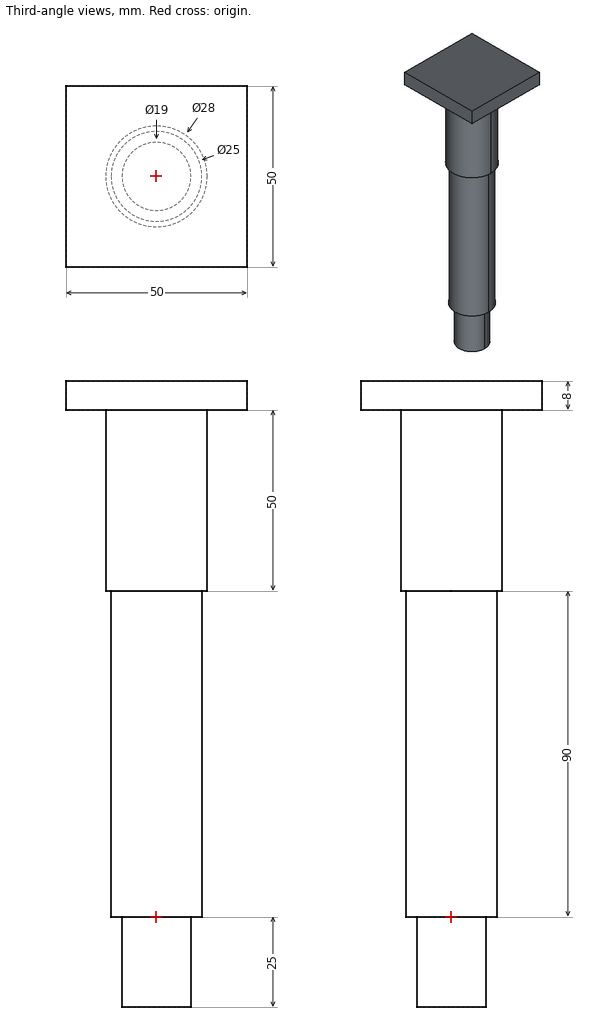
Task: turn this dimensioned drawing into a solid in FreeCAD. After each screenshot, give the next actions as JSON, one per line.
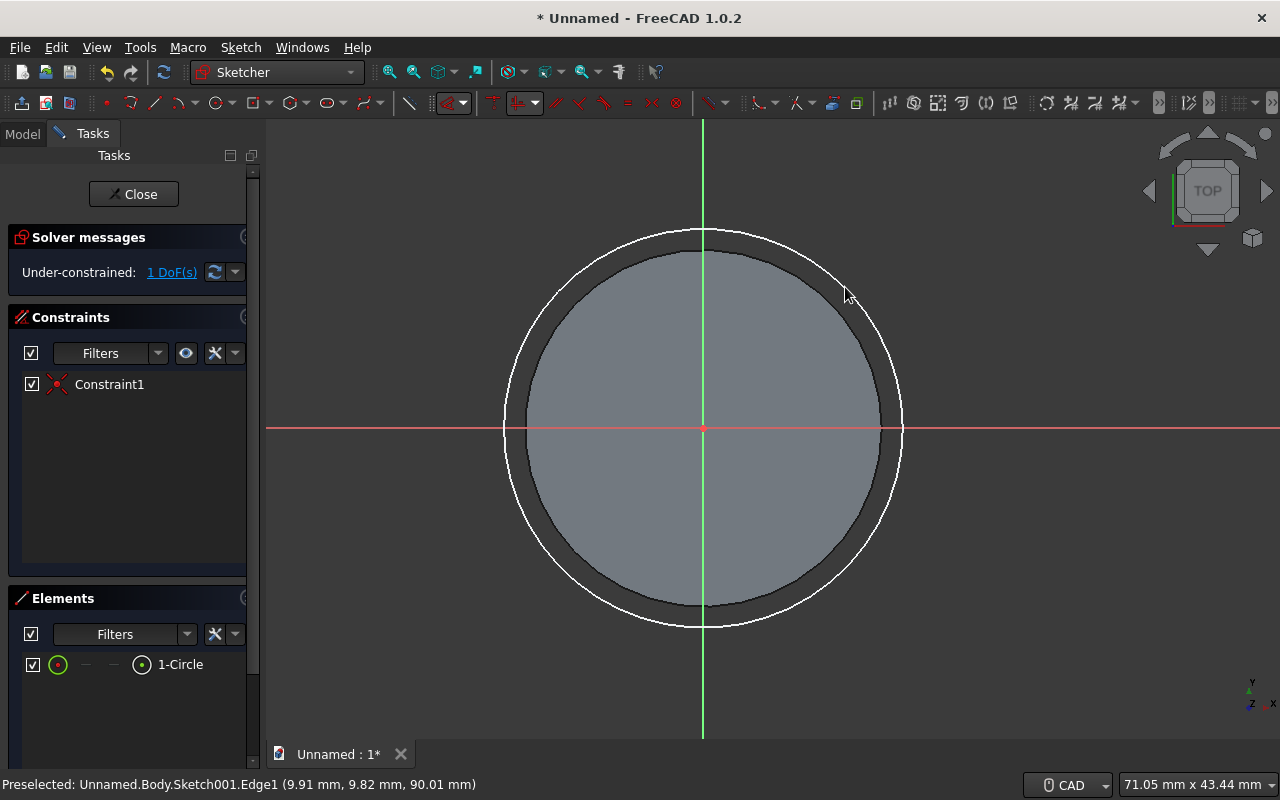
{"action": "key", "text": "d"}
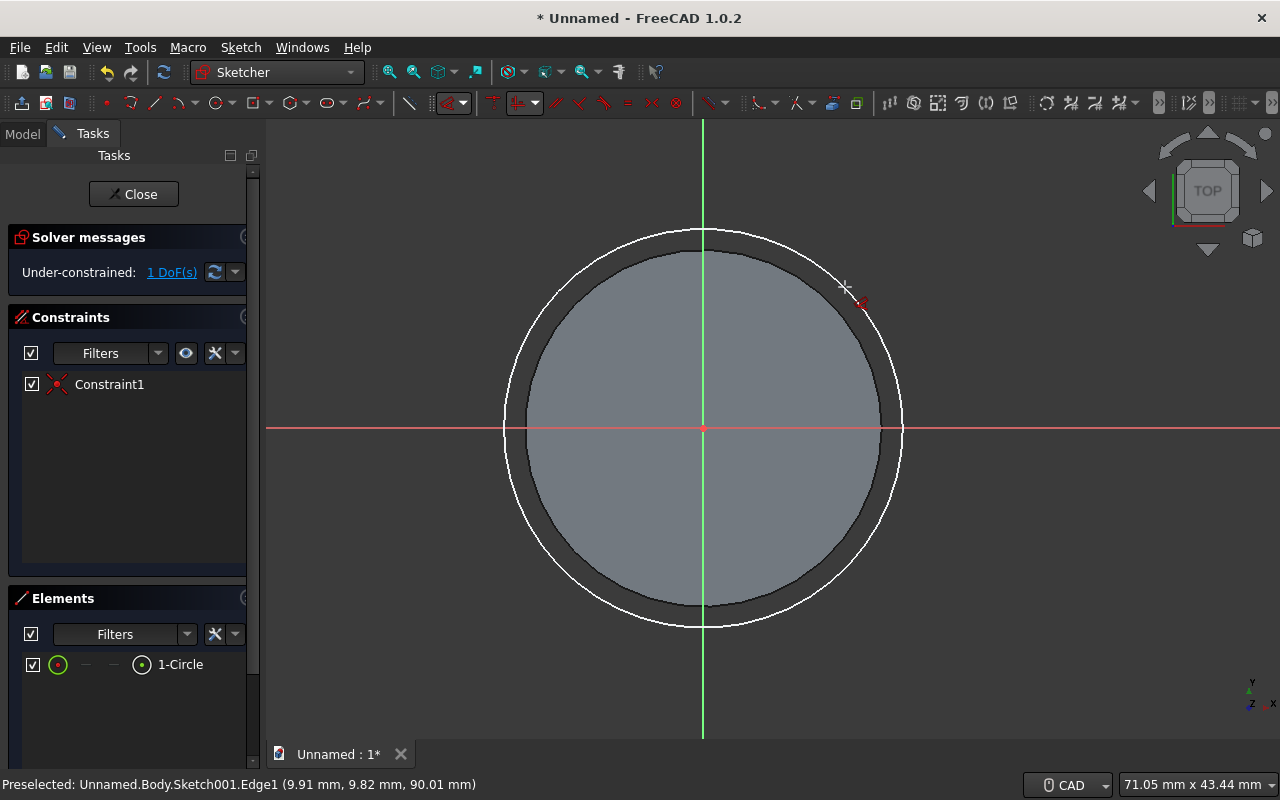
{"action": "left_click", "coordinate": [844, 287]}
{"action": "left_click", "coordinate": [867, 264]}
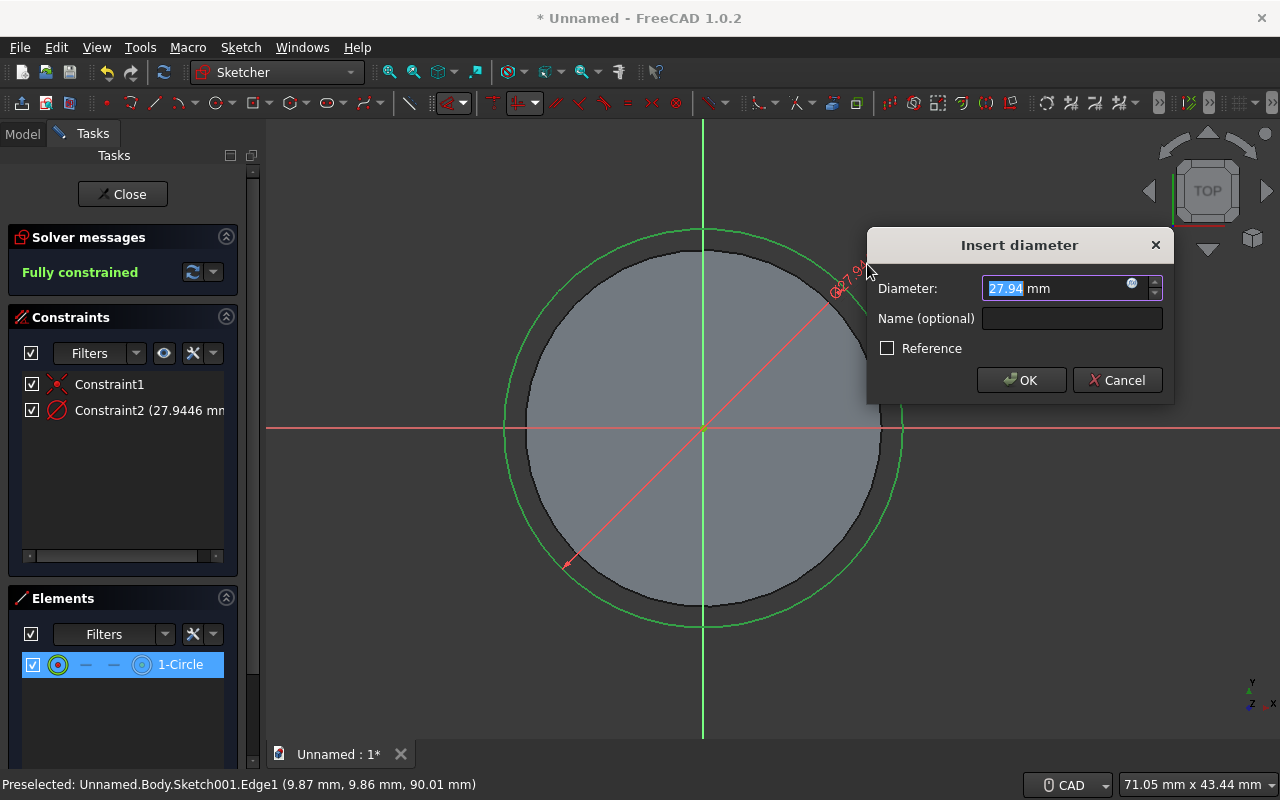
{"action": "type", "text": "28"}
{"action": "key", "text": "Return"}
{"action": "key", "text": "Escape"}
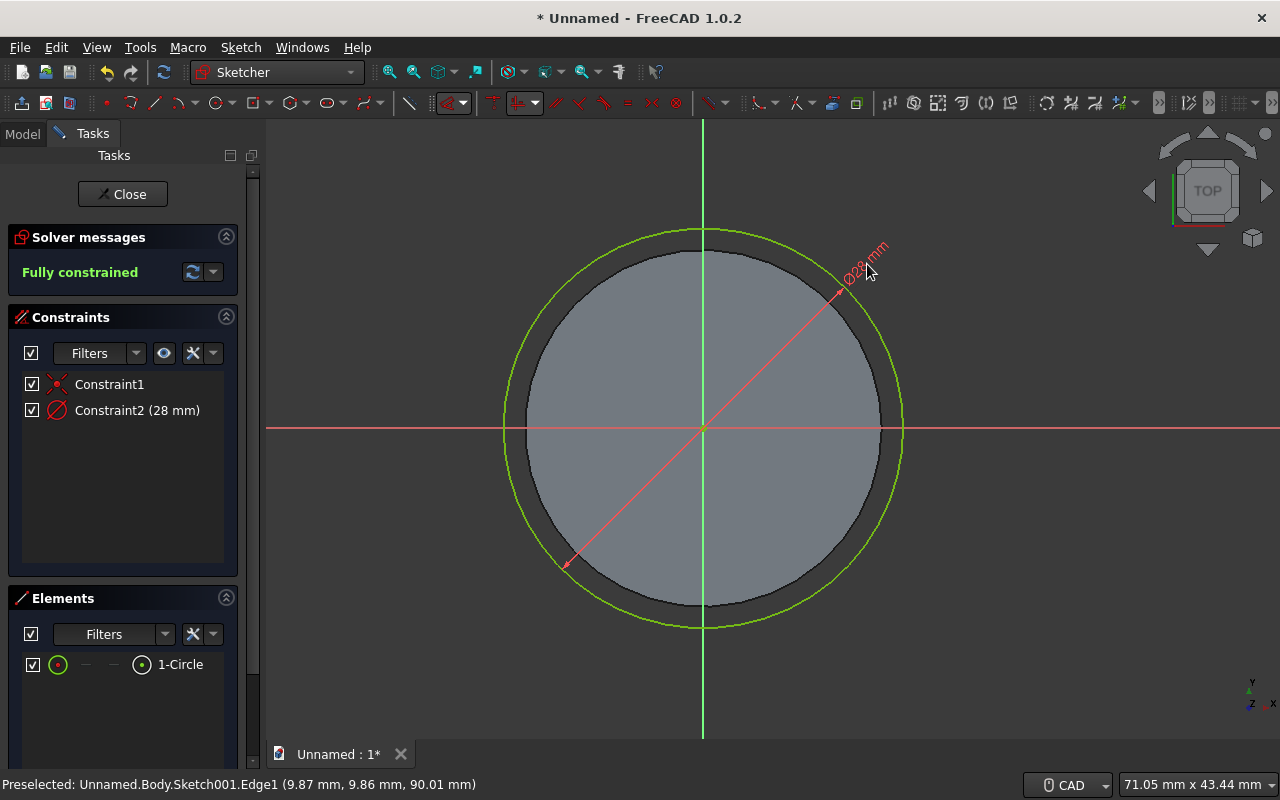
{"action": "left_click", "coordinate": [123, 194]}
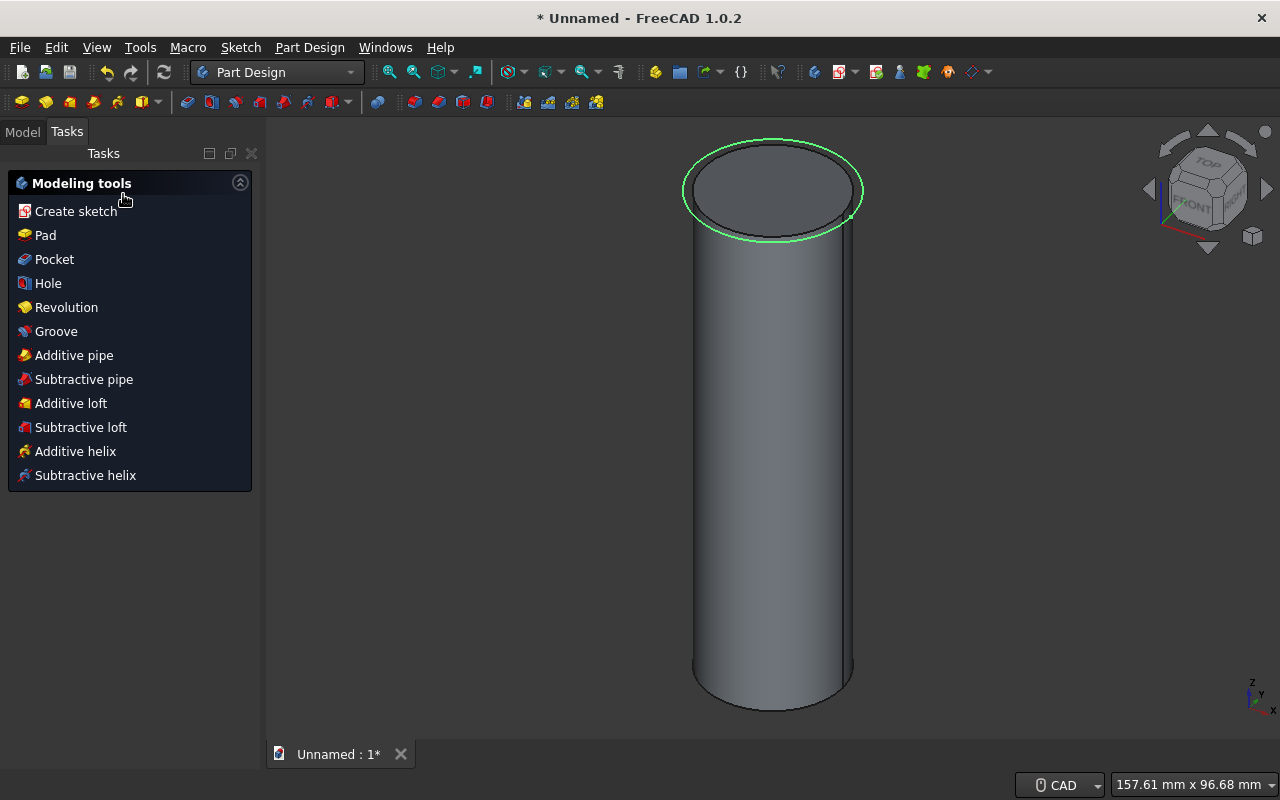
{"action": "left_click", "coordinate": [22, 102]}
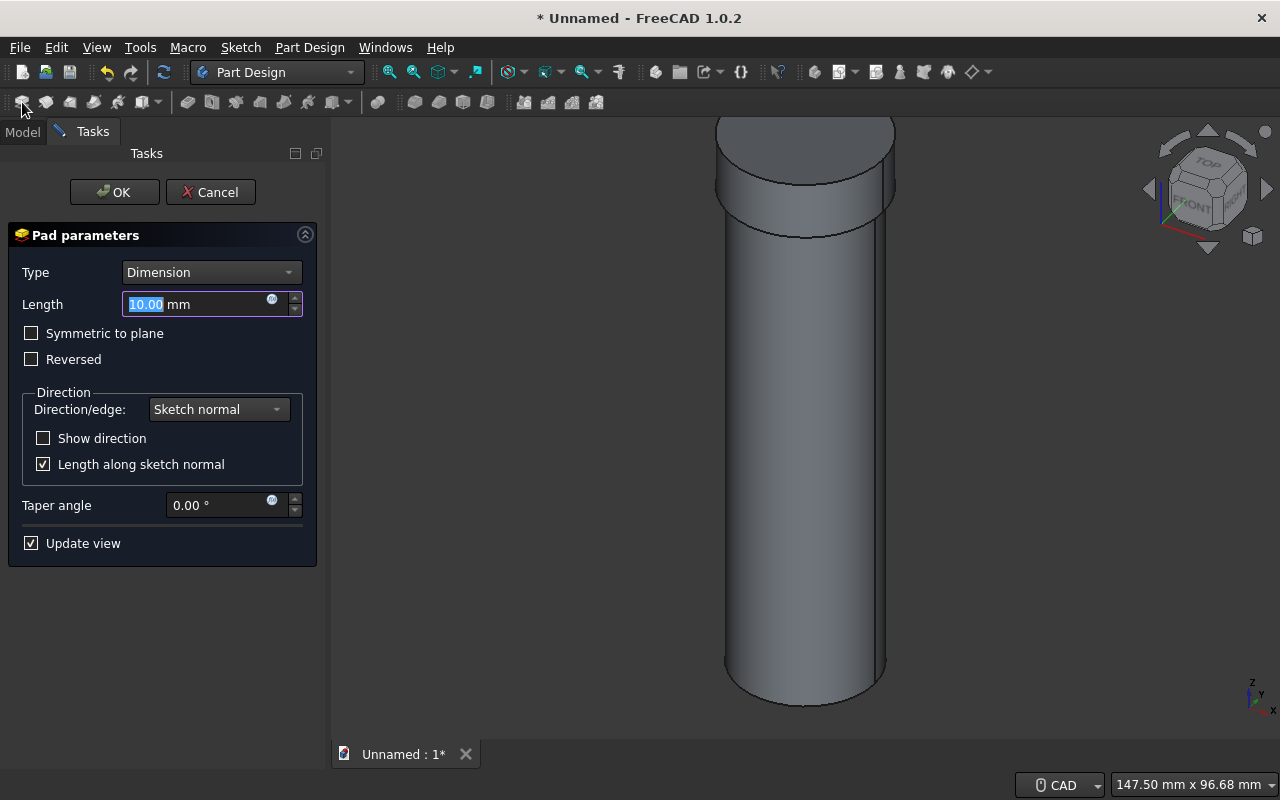
{"action": "type", "text": "50"}
{"action": "key", "text": "Tab"}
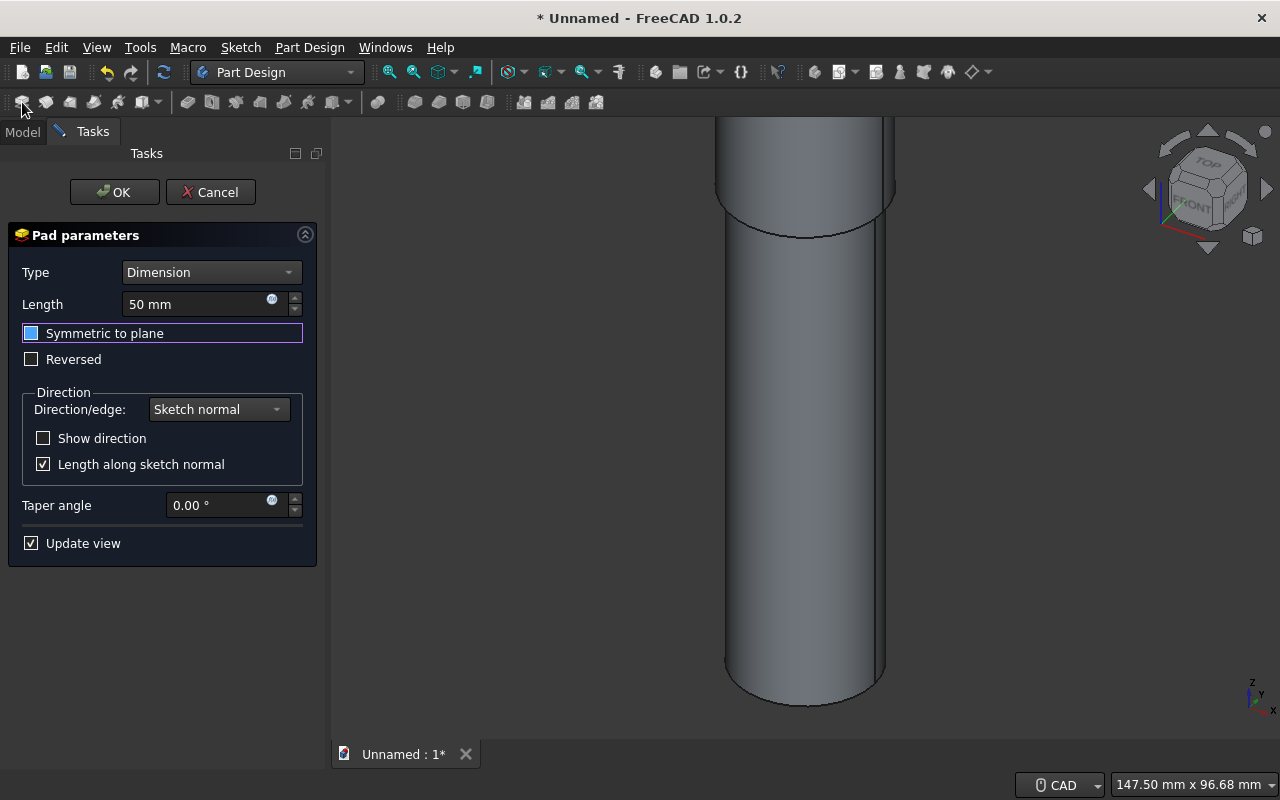
{"action": "left_click", "coordinate": [115, 192]}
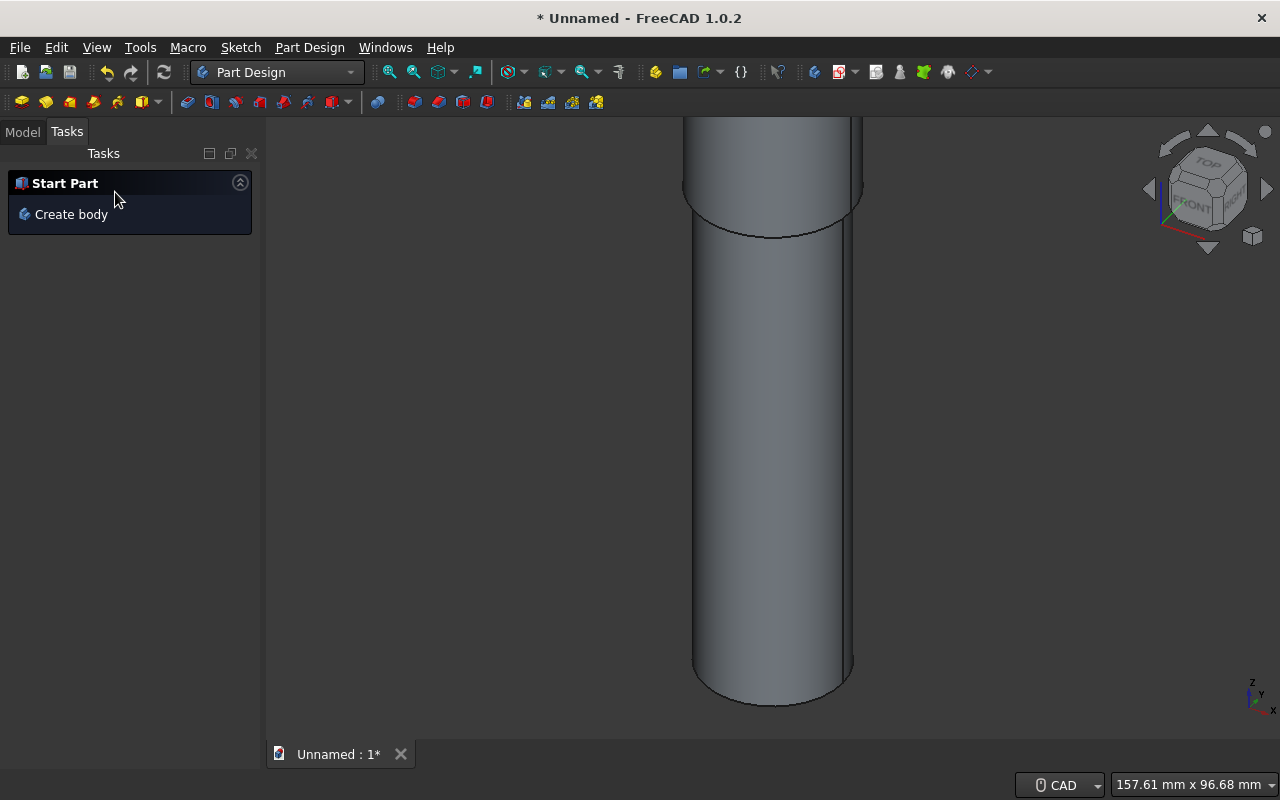
{"action": "key", "text": "v f"}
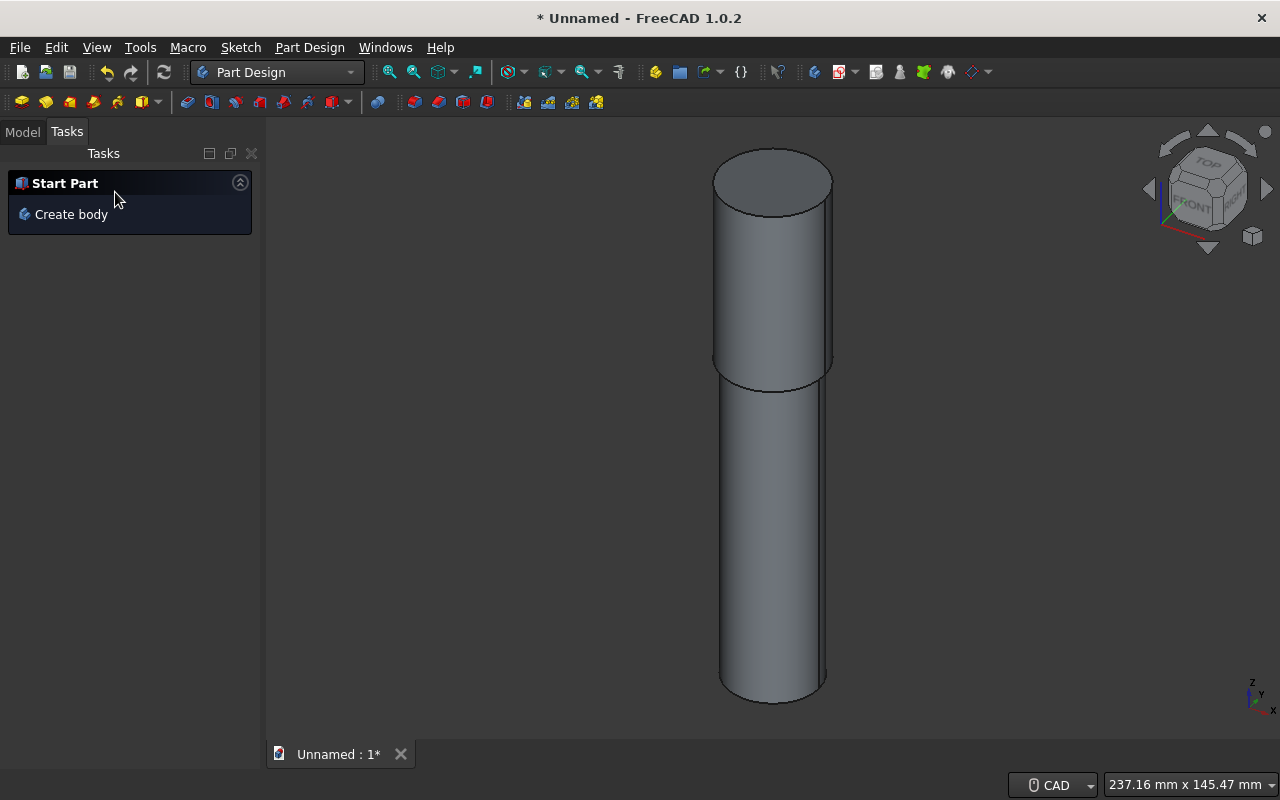
{"action": "left_click", "coordinate": [773, 182]}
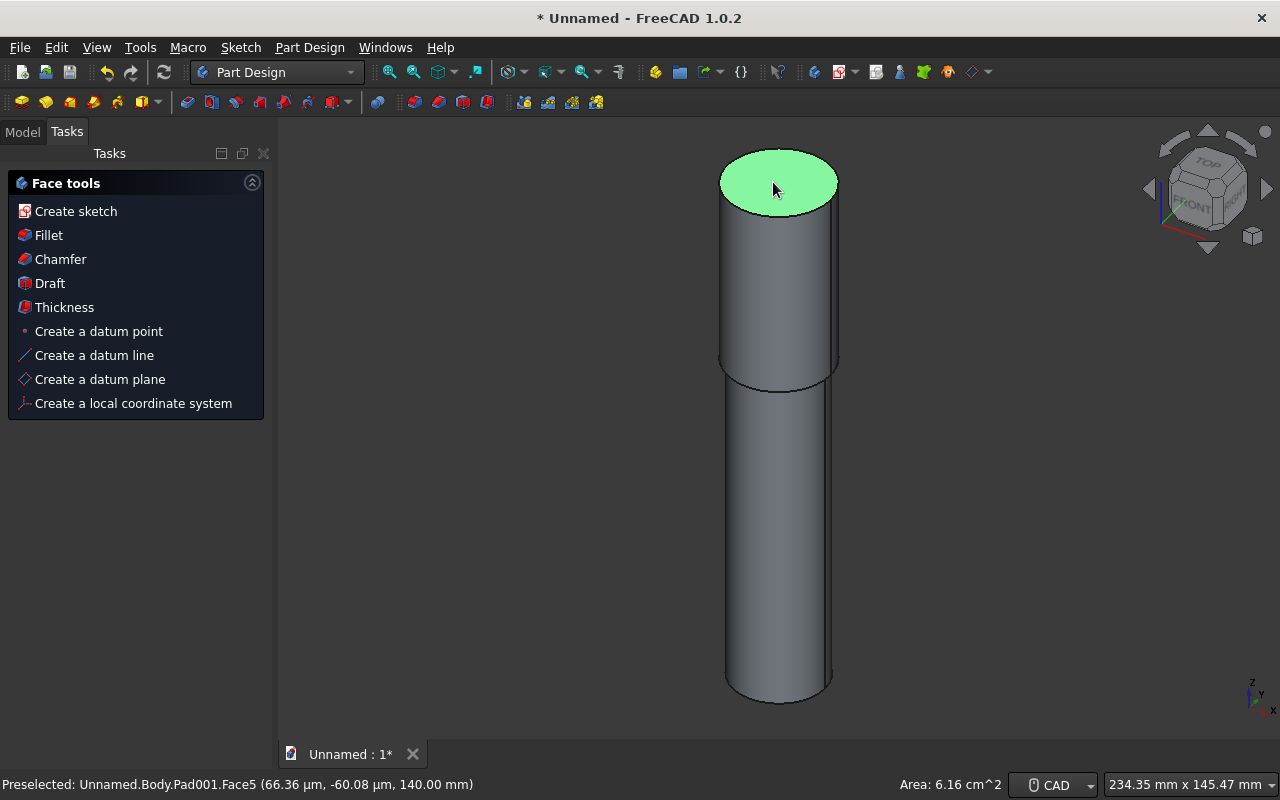
{"action": "left_click", "coordinate": [840, 72]}